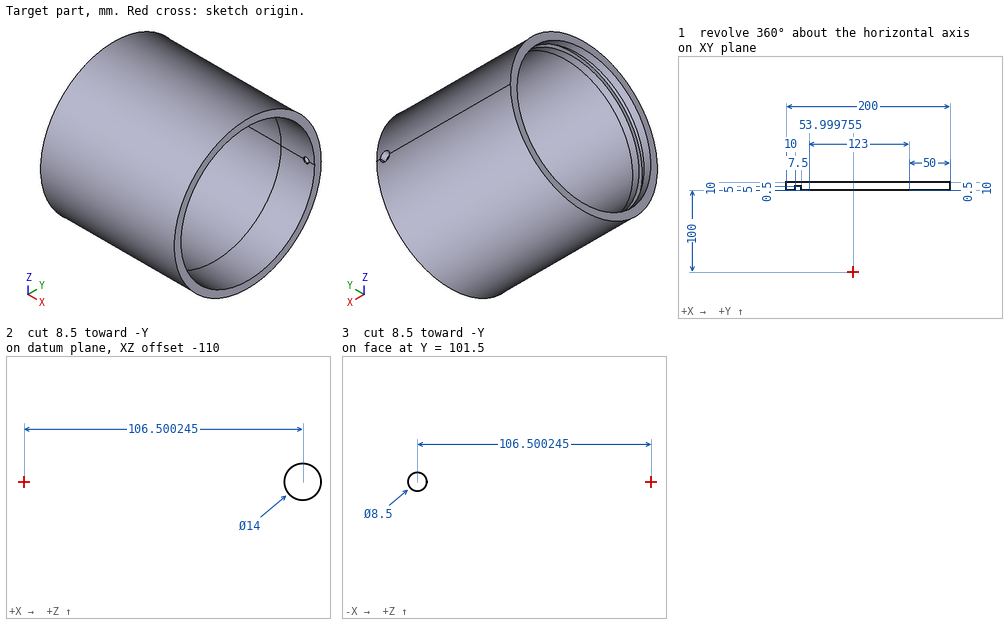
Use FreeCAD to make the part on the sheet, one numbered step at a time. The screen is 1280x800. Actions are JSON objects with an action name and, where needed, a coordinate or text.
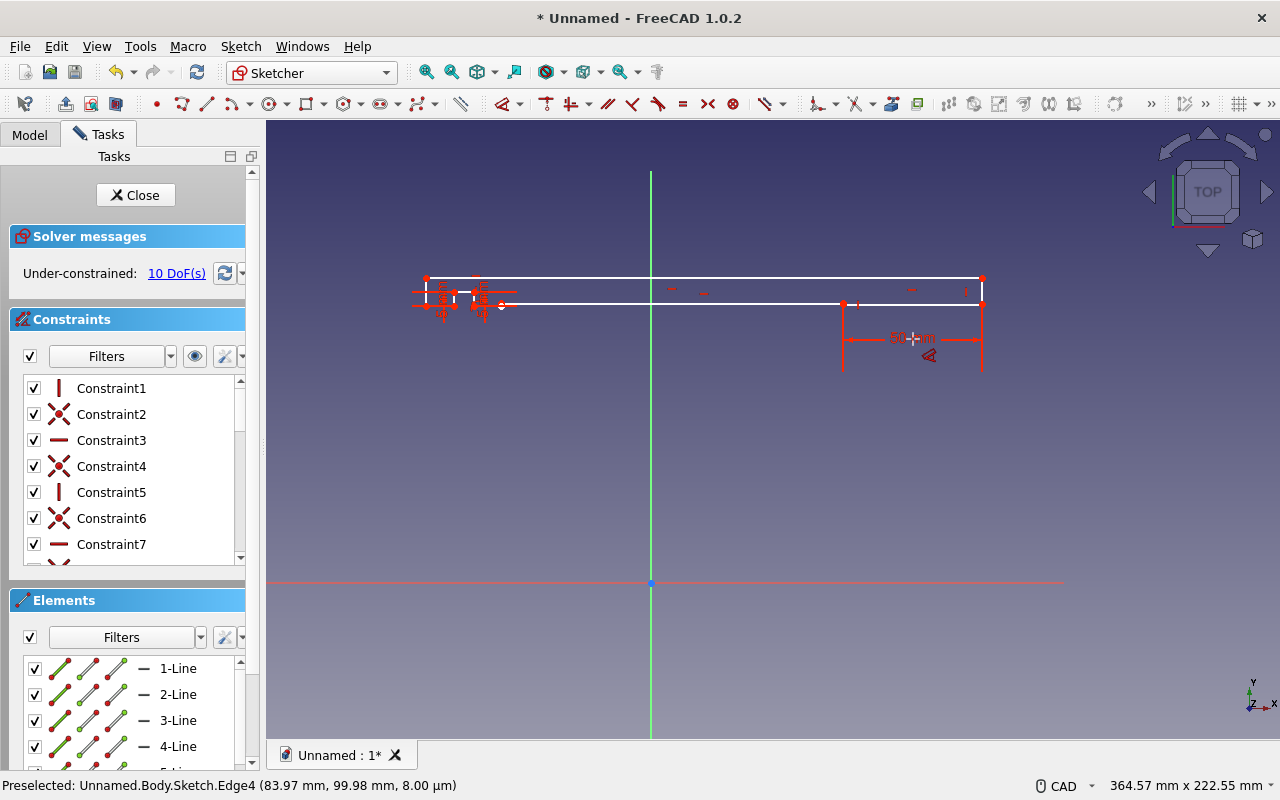
{"action": "scroll", "coordinate": [982, 294], "scroll_direction": "up", "scroll_amount": 2}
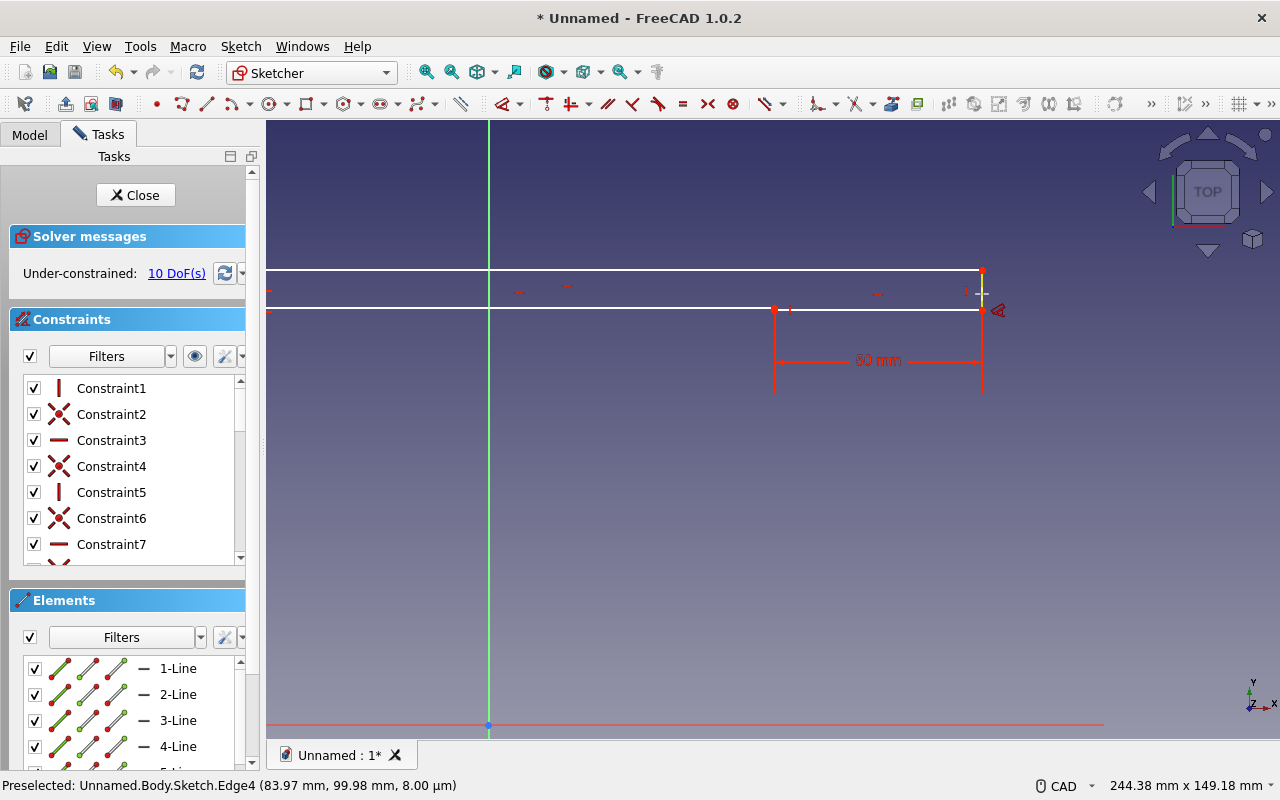
{"action": "left_click", "coordinate": [982, 294]}
{"action": "left_click", "coordinate": [1016, 290]}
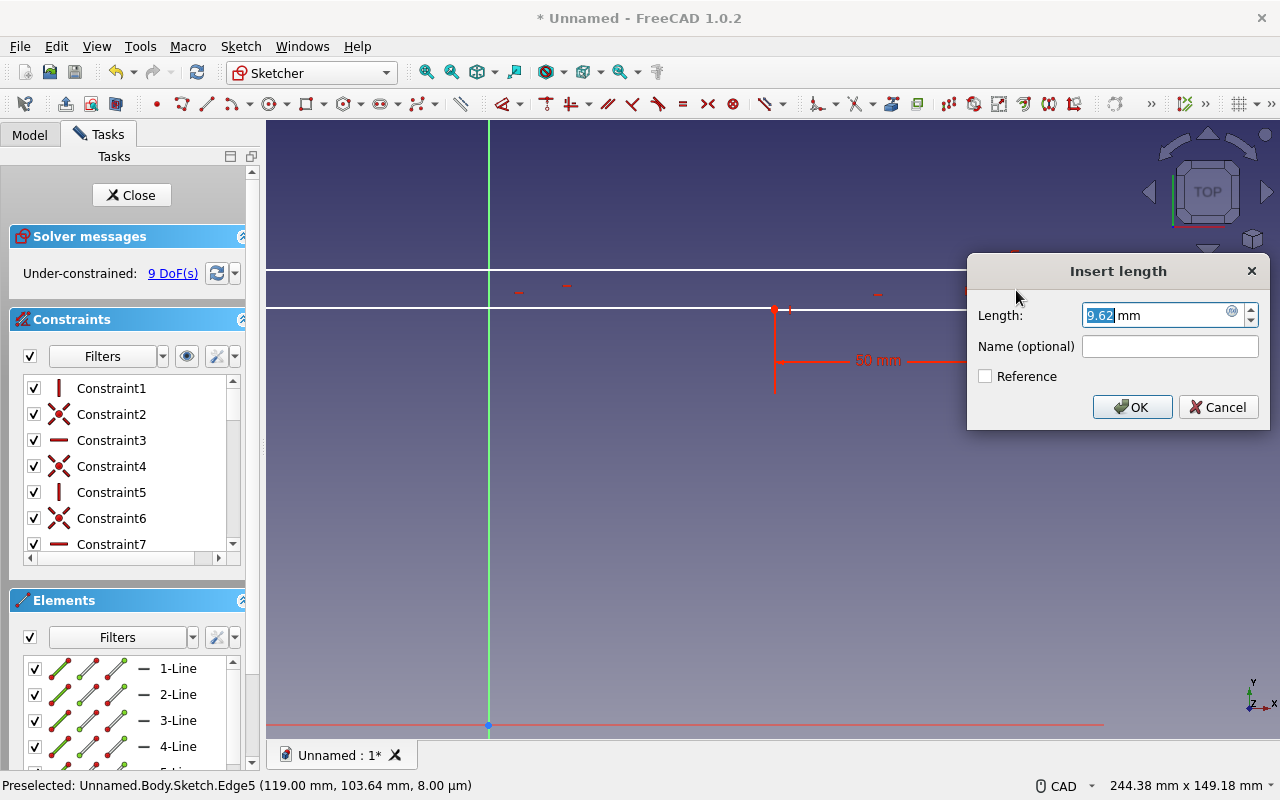
{"action": "type", "text": "10"}
{"action": "key", "text": "Return"}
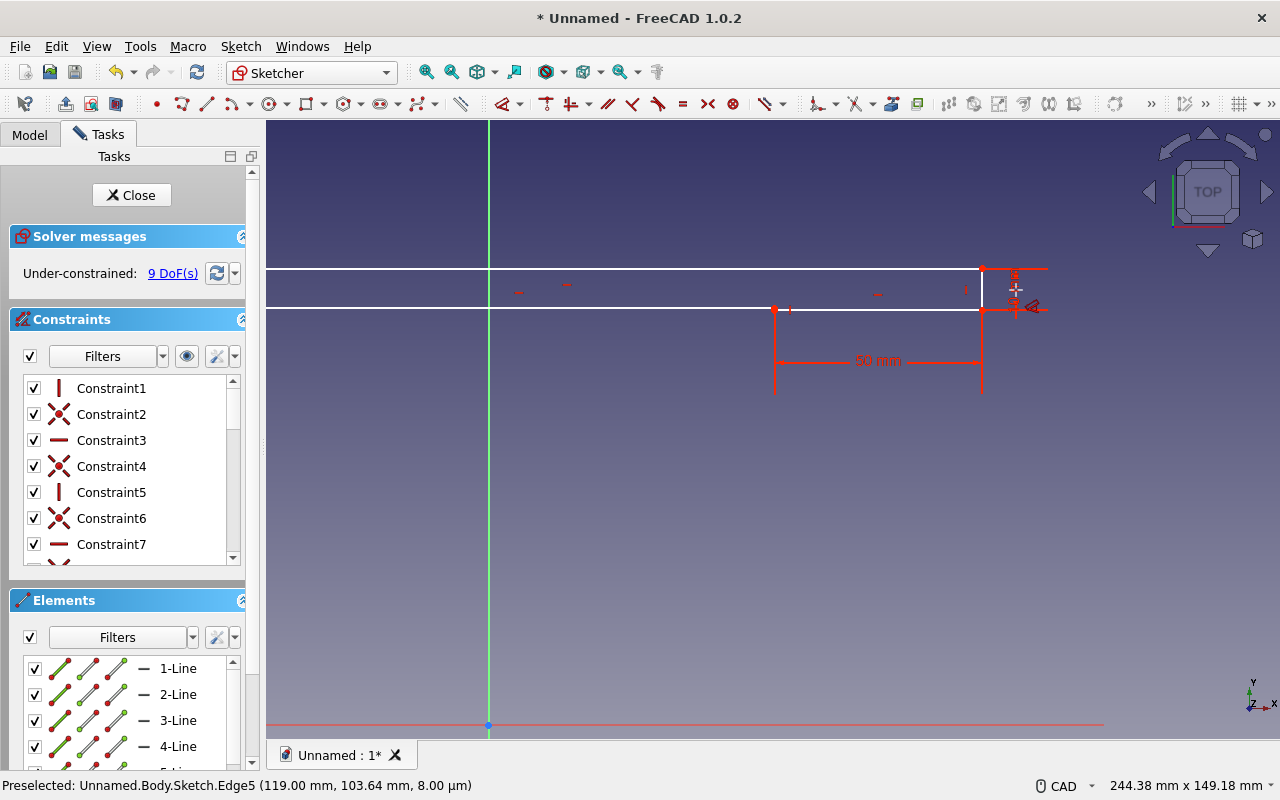
{"action": "scroll", "coordinate": [983, 293], "scroll_direction": "down", "scroll_amount": 2}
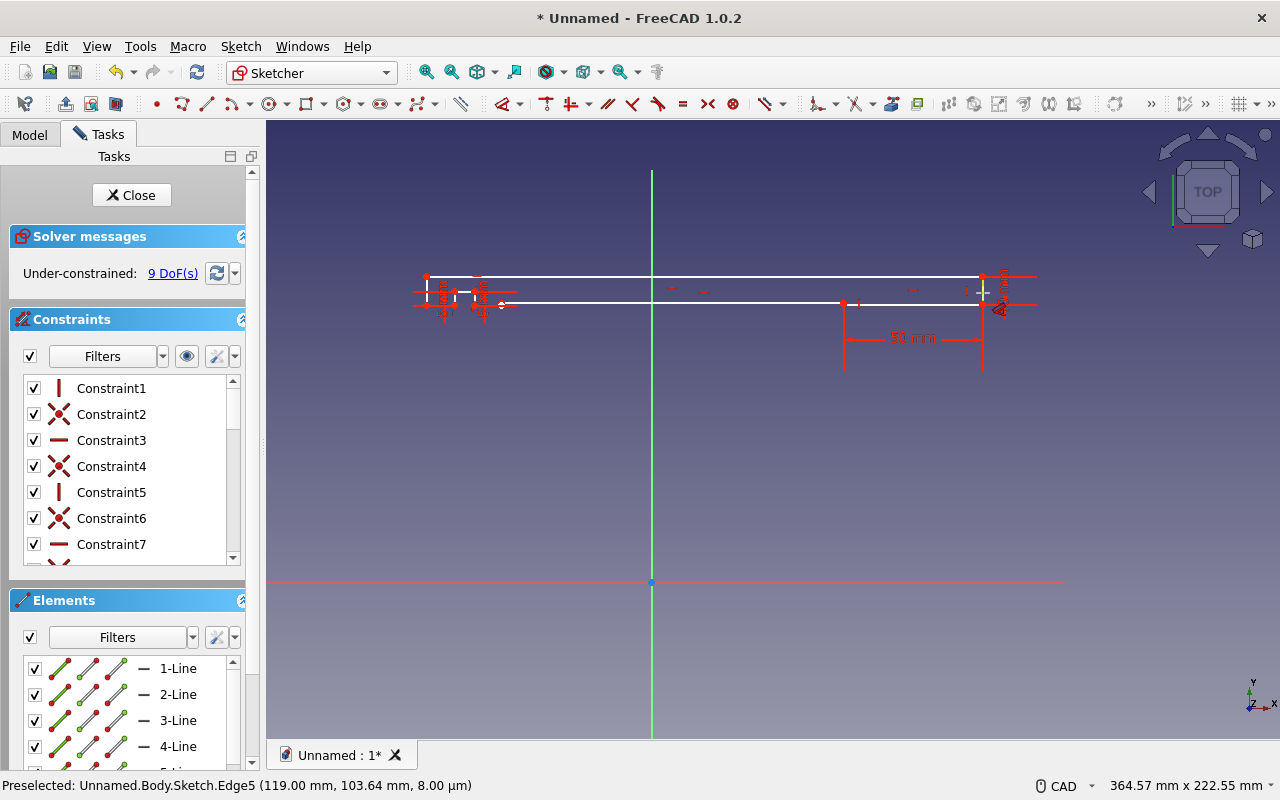
{"action": "scroll", "coordinate": [427, 286], "scroll_direction": "up", "scroll_amount": 3}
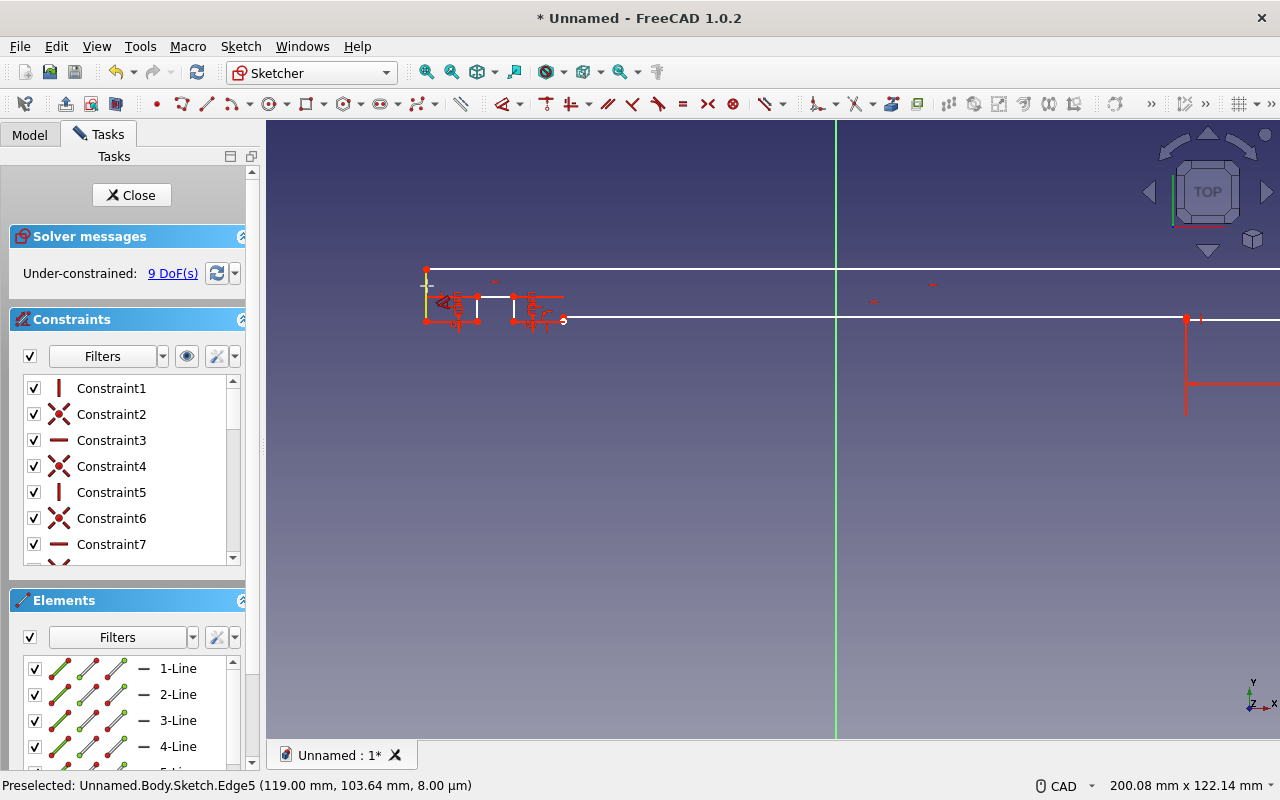
{"action": "left_click", "coordinate": [426, 285]}
{"action": "left_click", "coordinate": [392, 284]}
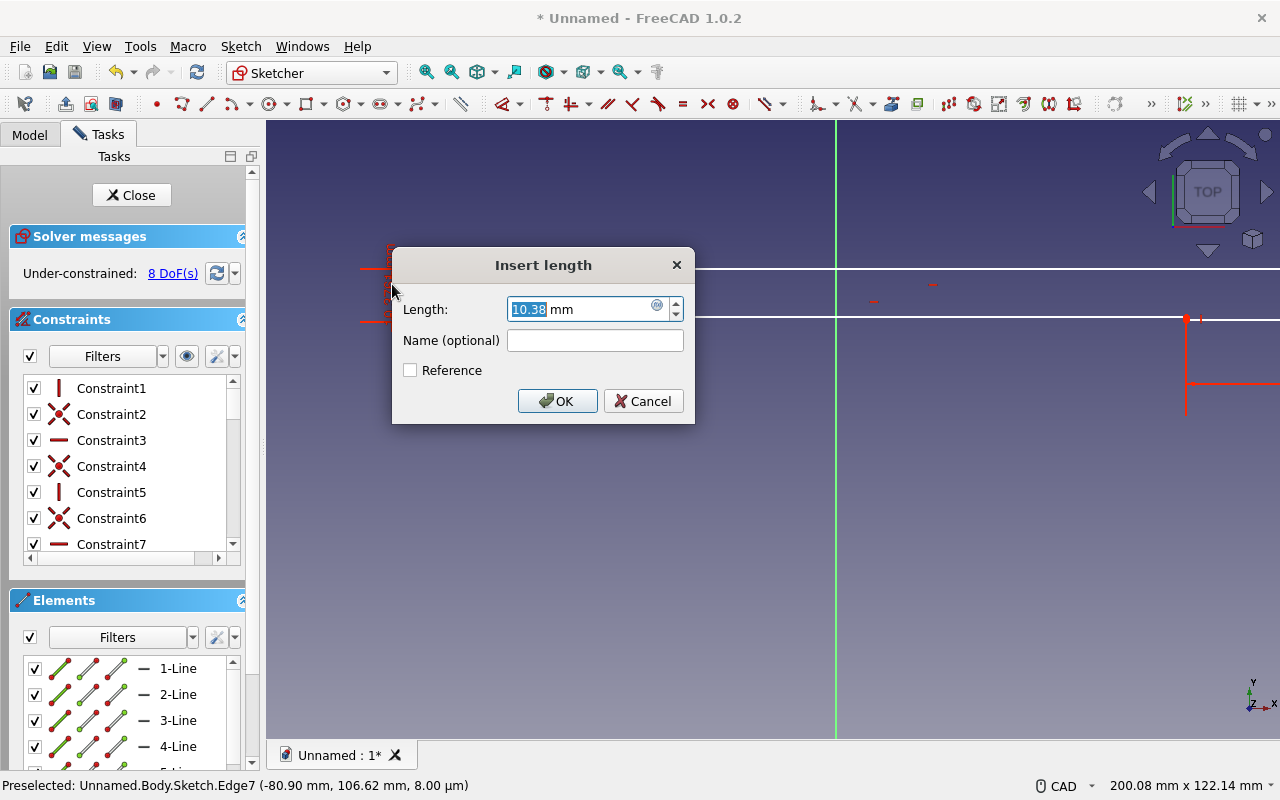
{"action": "type", "text": "10"}
{"action": "key", "text": "Return"}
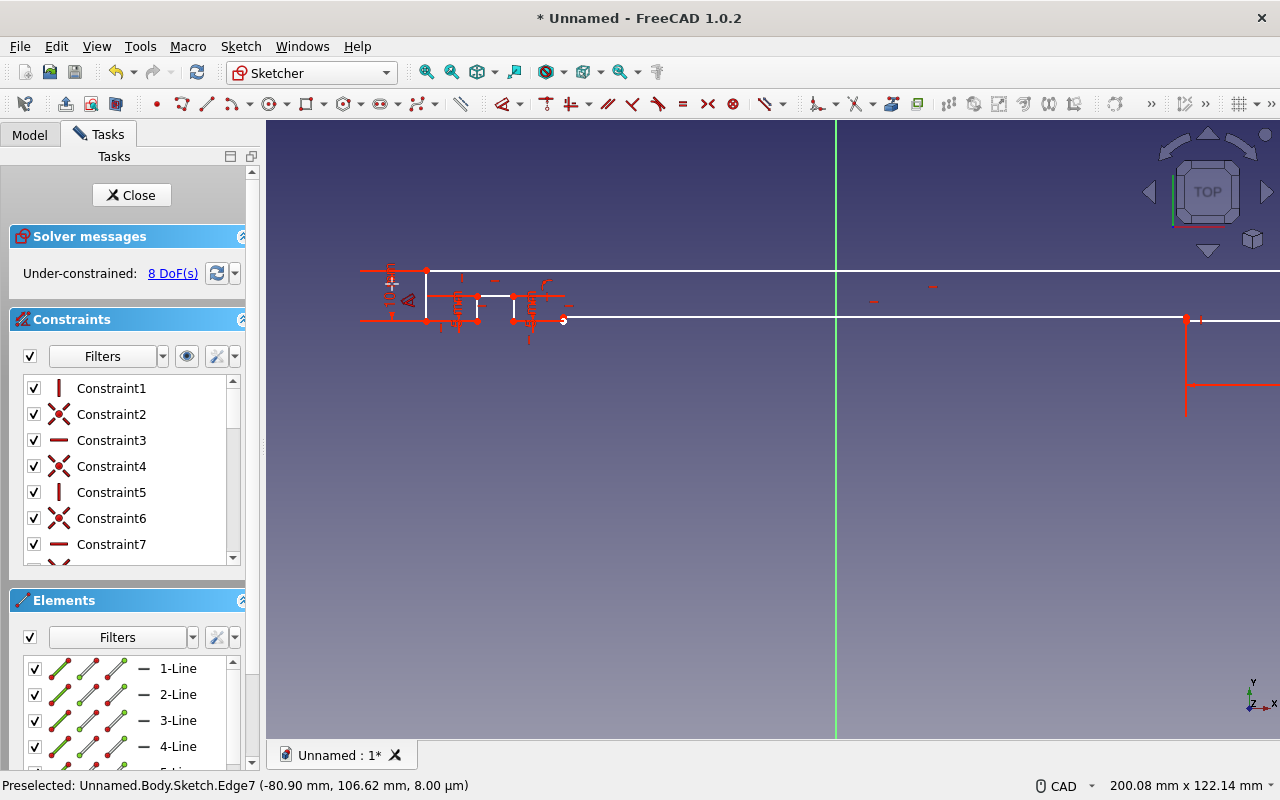
{"action": "left_click", "coordinate": [442, 321]}
{"action": "left_click", "coordinate": [464, 287]}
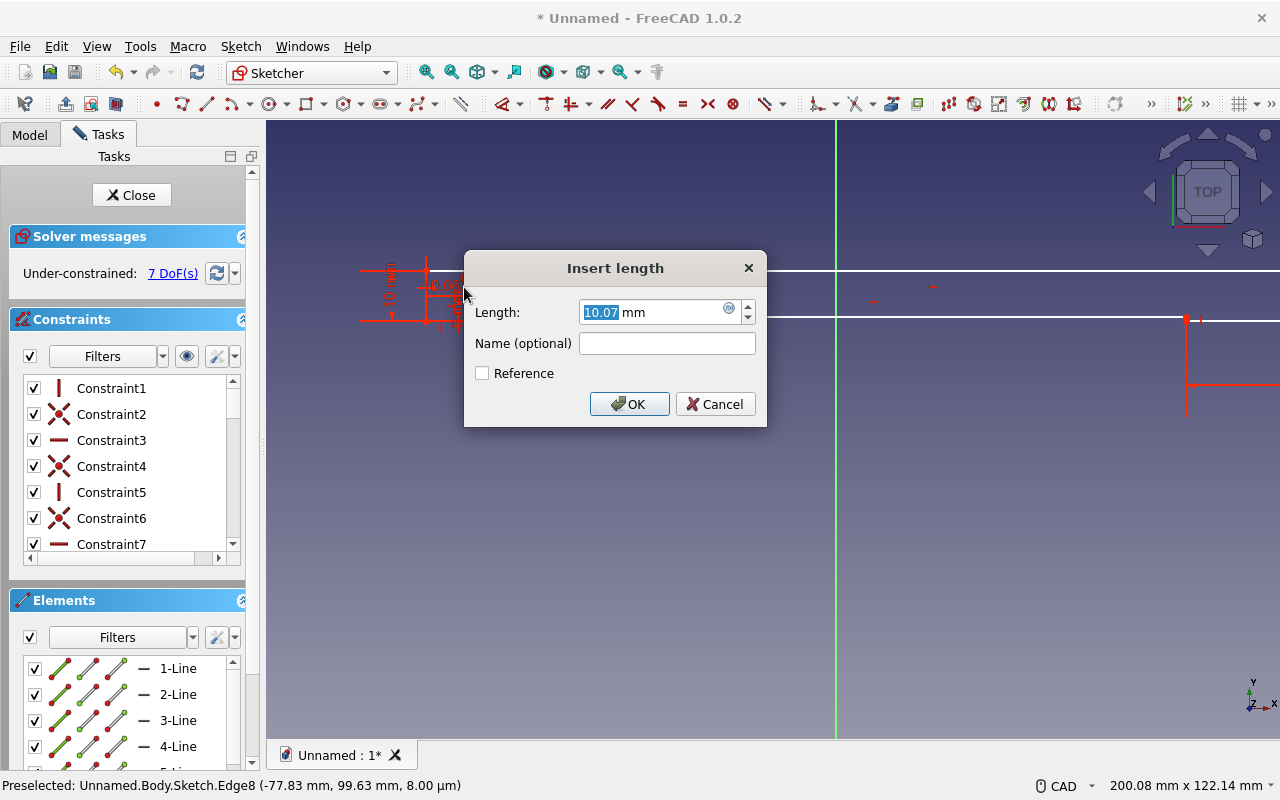
{"action": "type", "text": "10"}
{"action": "key", "text": "Return"}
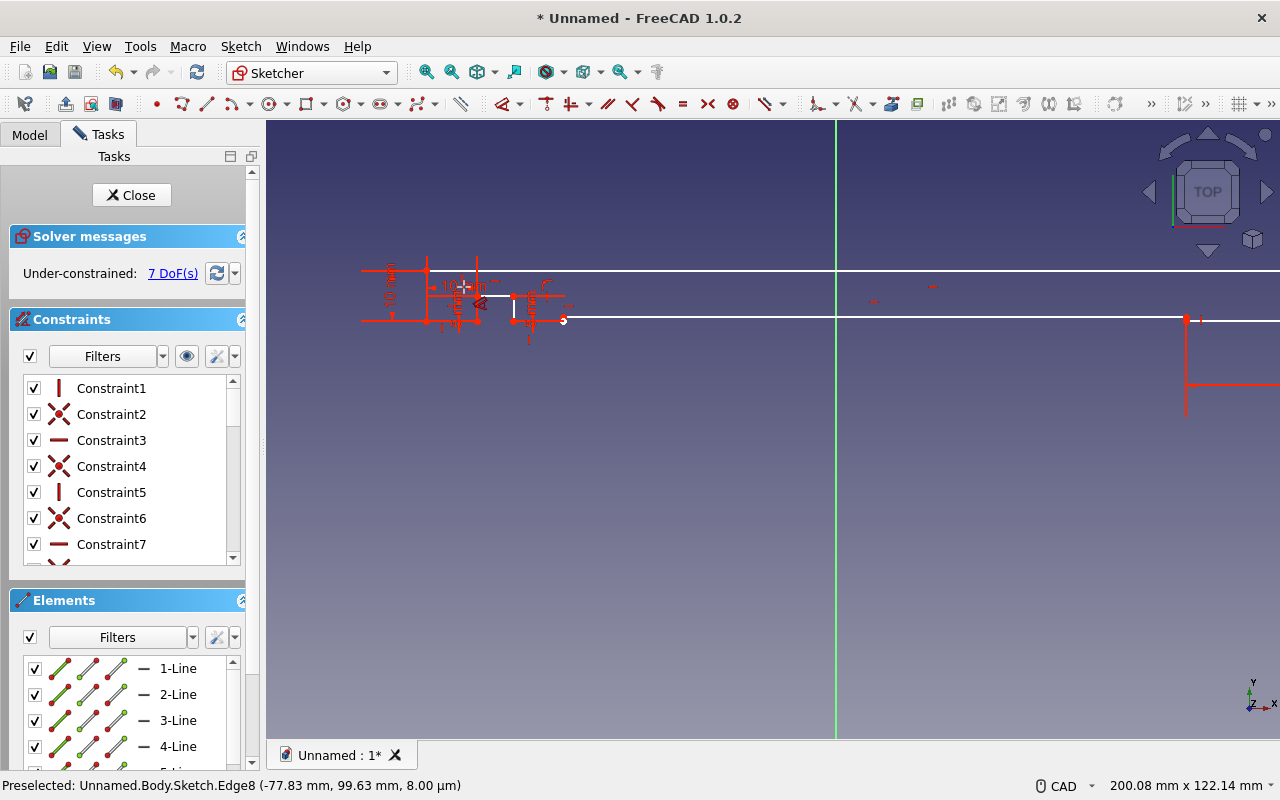
{"action": "scroll", "coordinate": [563, 319], "scroll_direction": "up", "scroll_amount": 14}